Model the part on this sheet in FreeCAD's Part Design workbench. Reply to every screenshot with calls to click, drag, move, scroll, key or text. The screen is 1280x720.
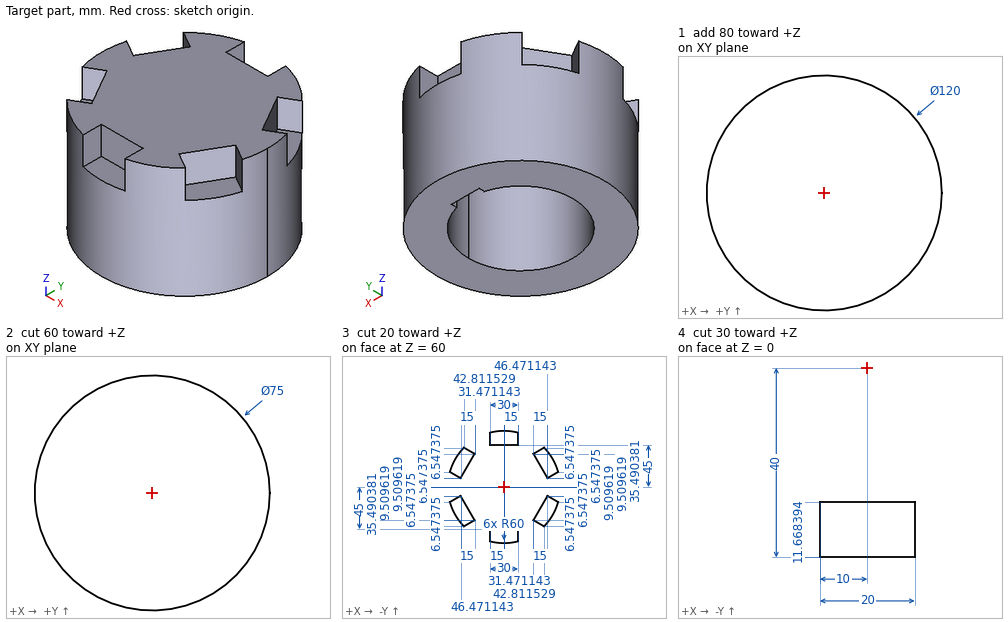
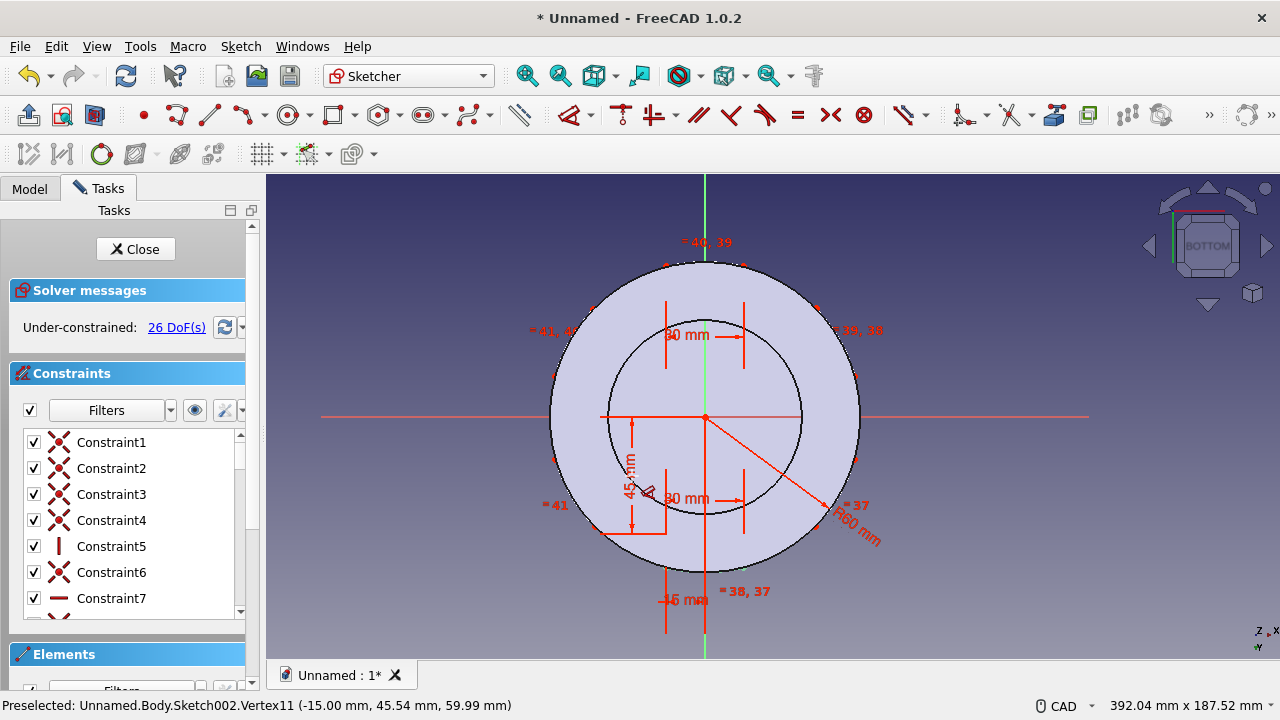
click(744, 267)
click(724, 233)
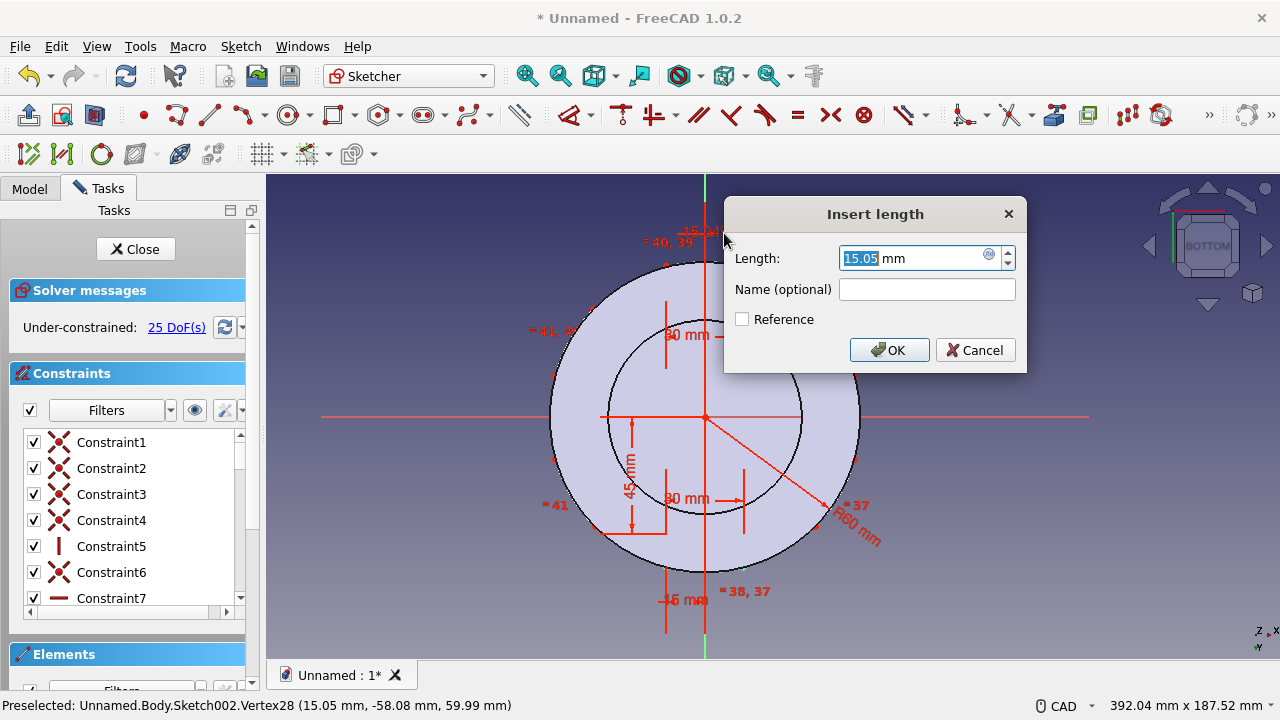
text(15)
key(Return)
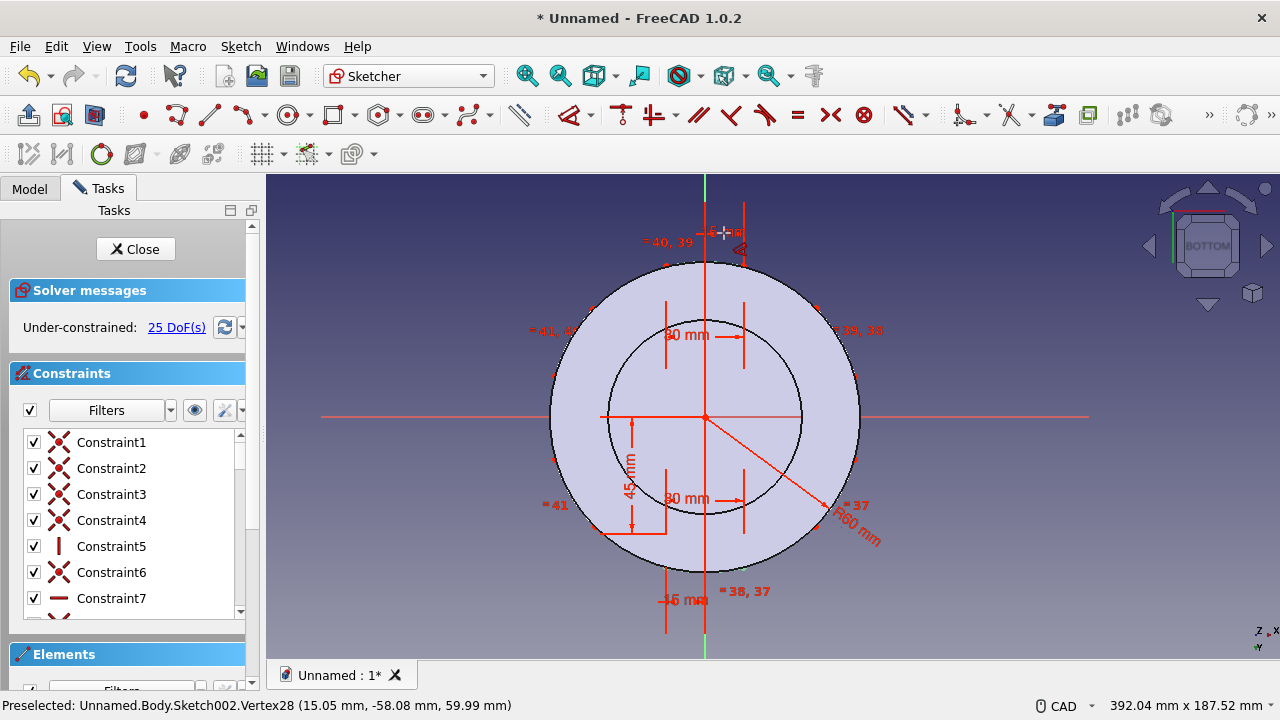
click(744, 302)
click(778, 359)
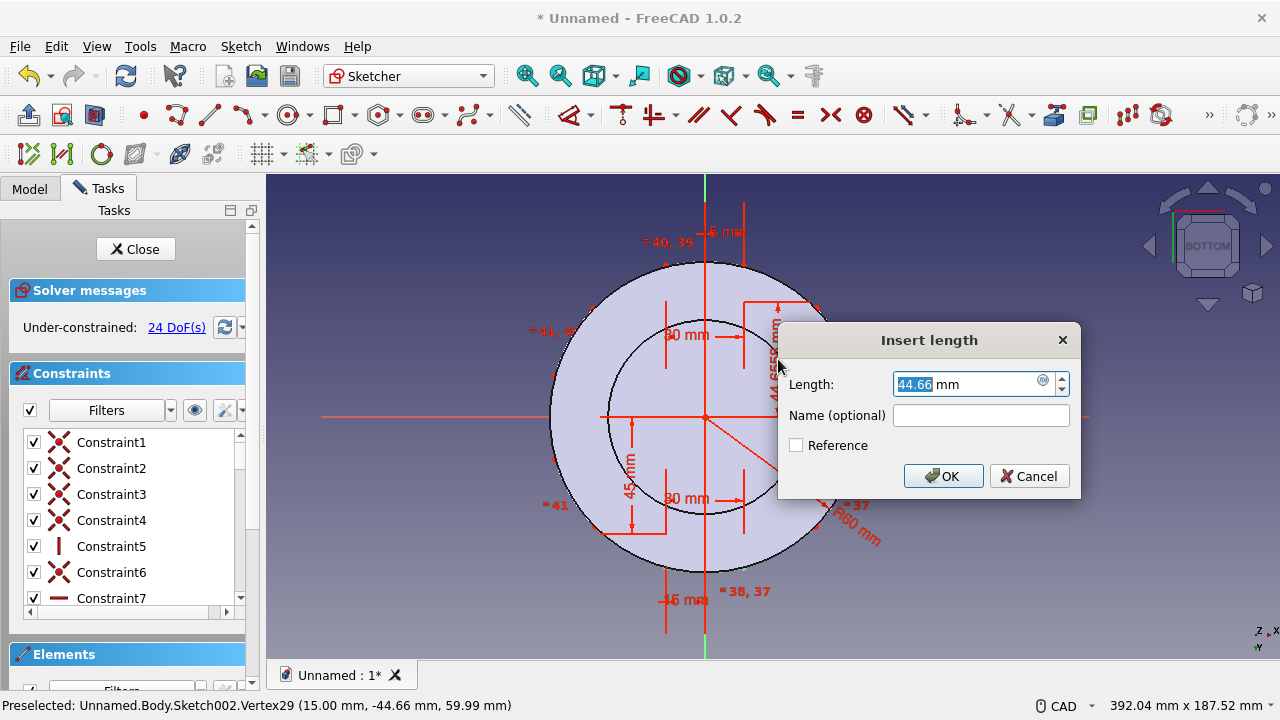
text(45)
key(Return)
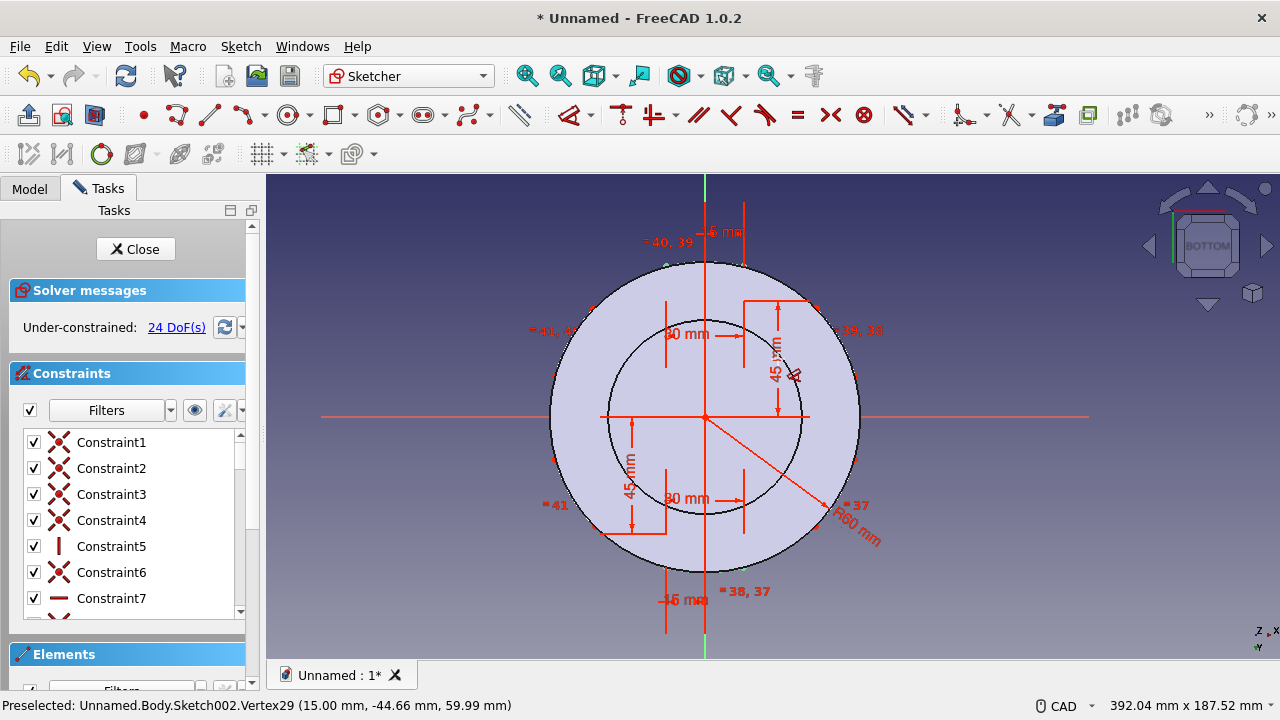
click(798, 490)
click(806, 568)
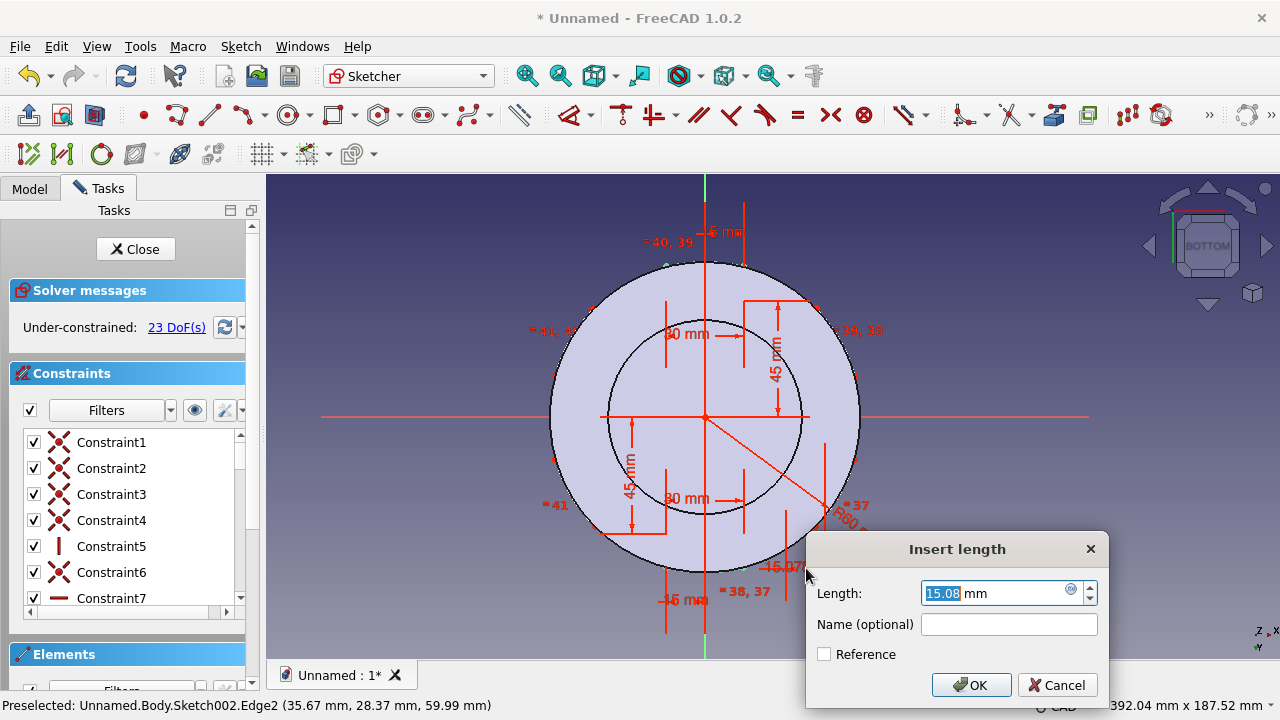
text(15)
key(Return)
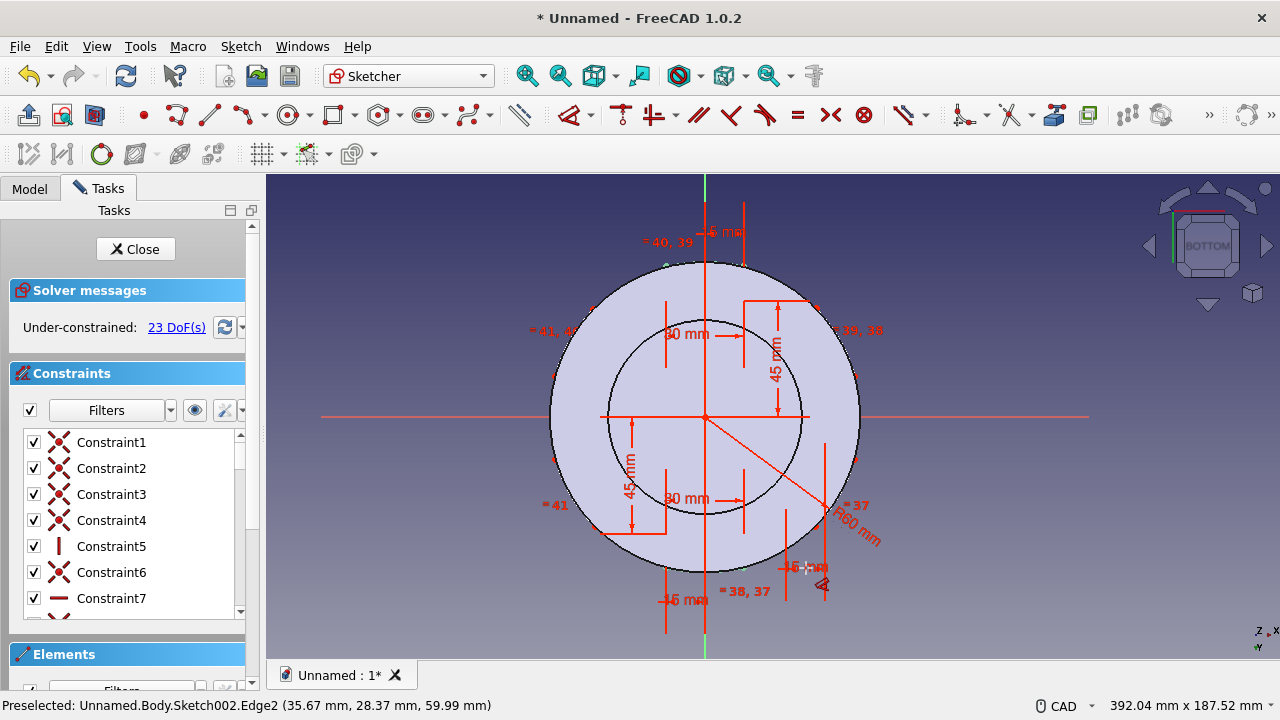
click(813, 374)
click(805, 292)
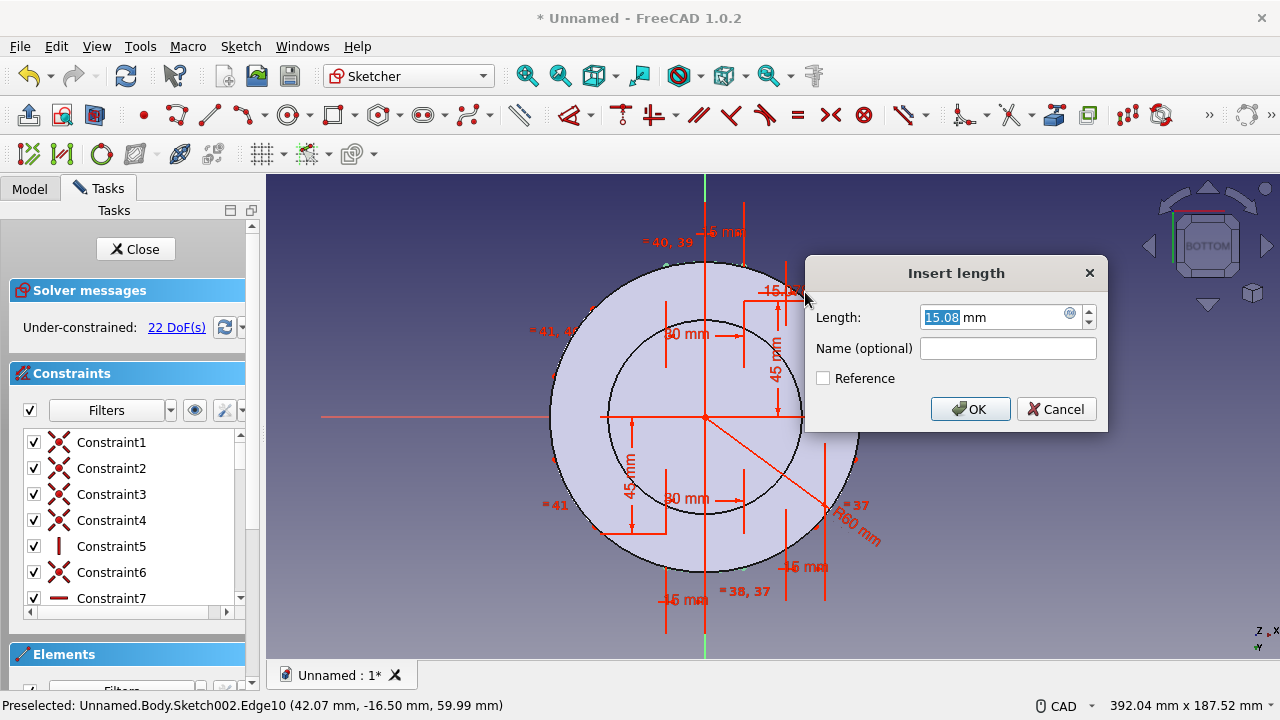
text(15)
key(Return)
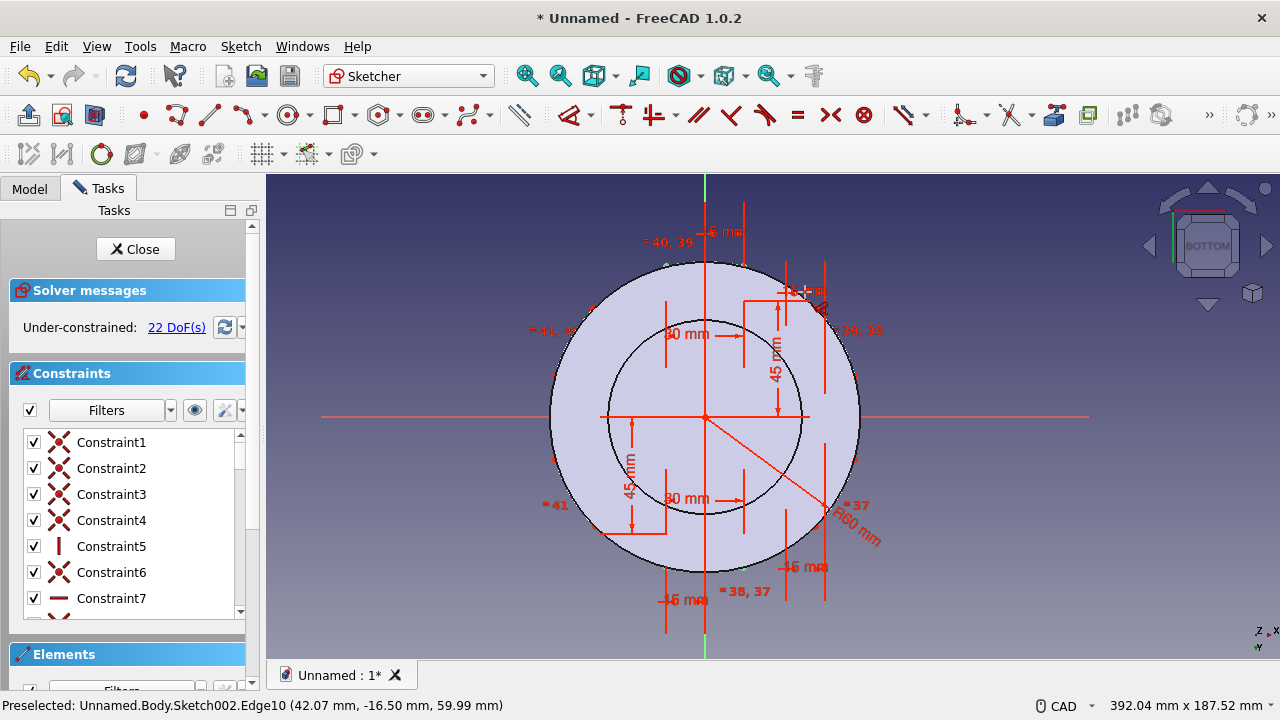
click(612, 347)
click(604, 293)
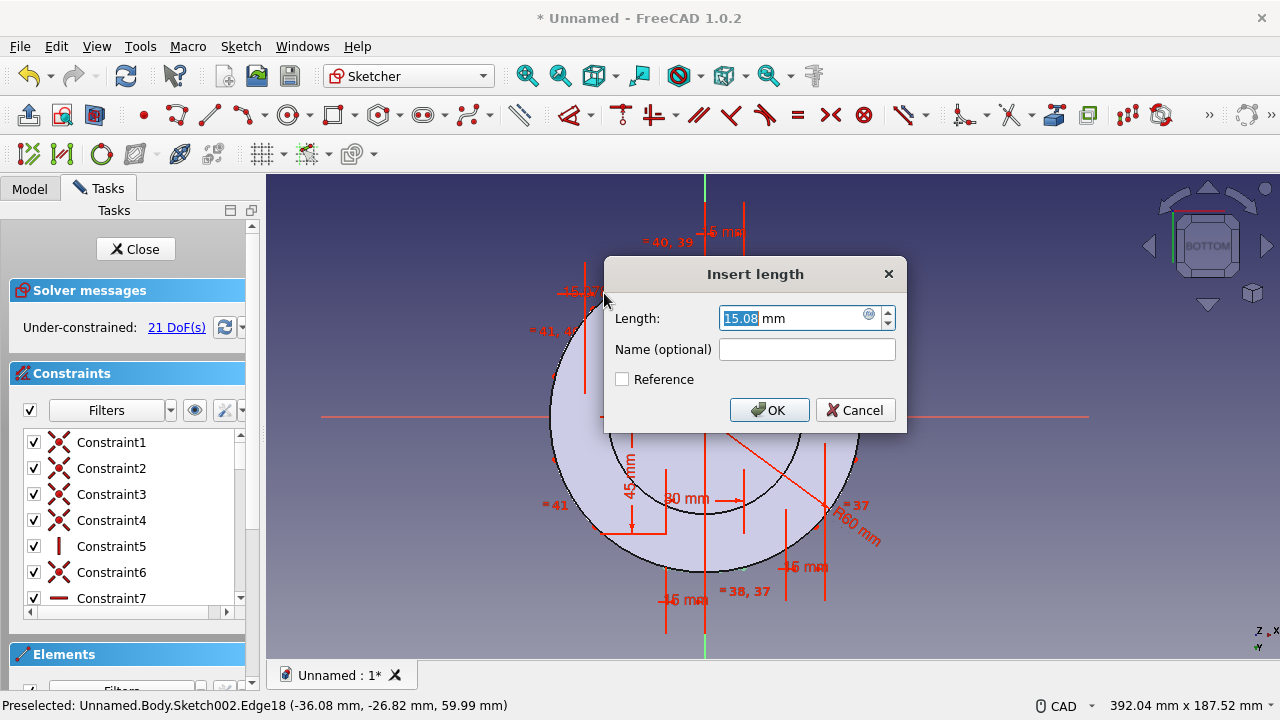
text(15)
key(Return)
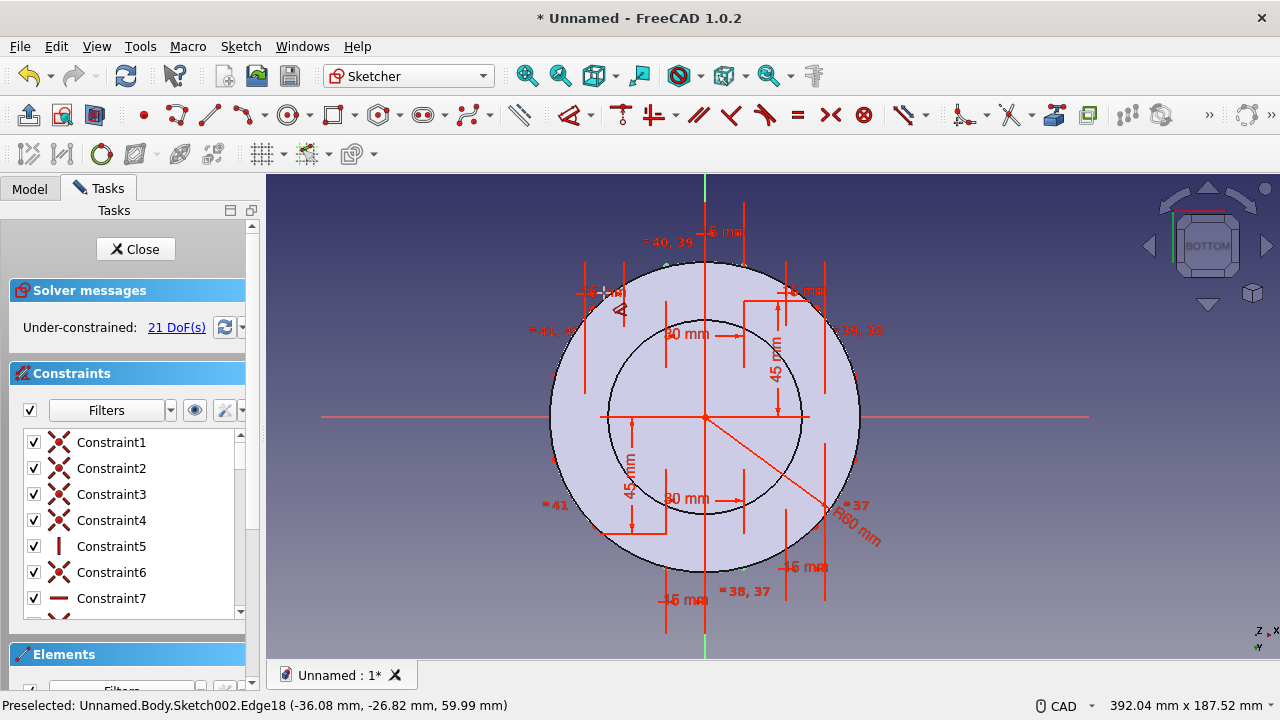
click(597, 463)
click(604, 544)